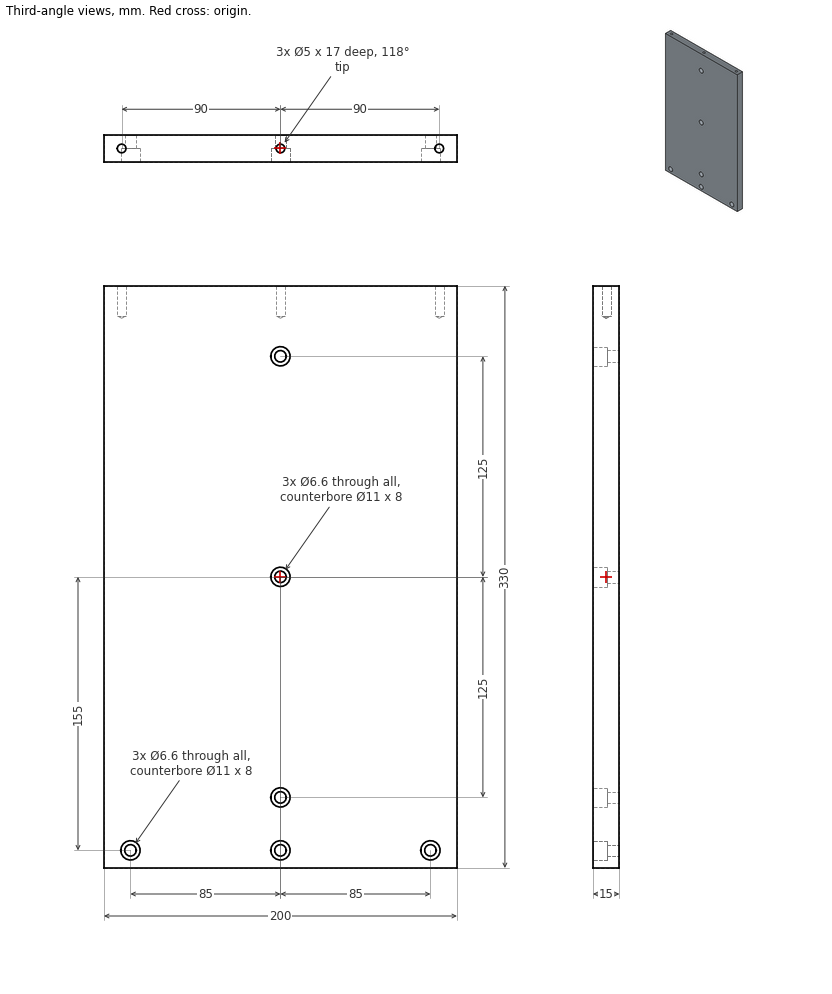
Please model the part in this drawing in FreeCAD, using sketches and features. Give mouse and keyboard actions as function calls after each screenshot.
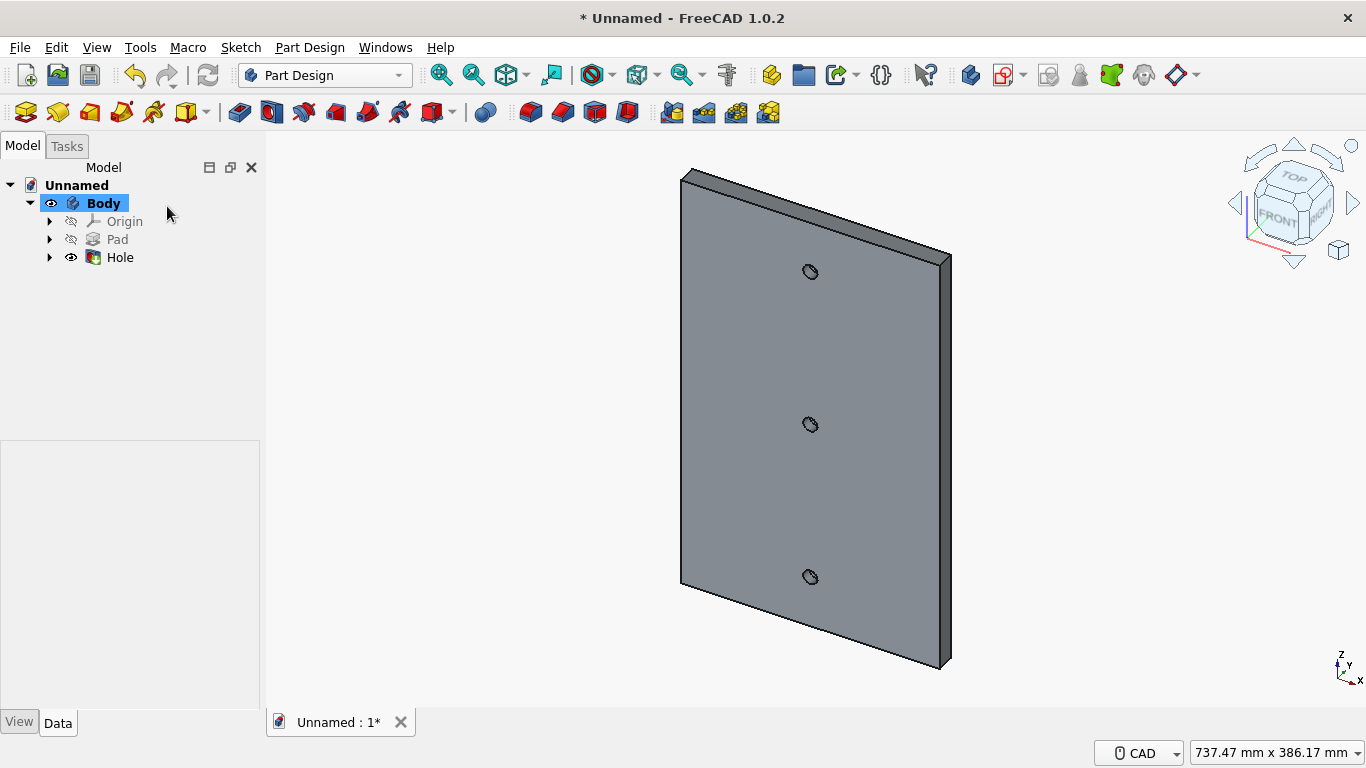
click(847, 493)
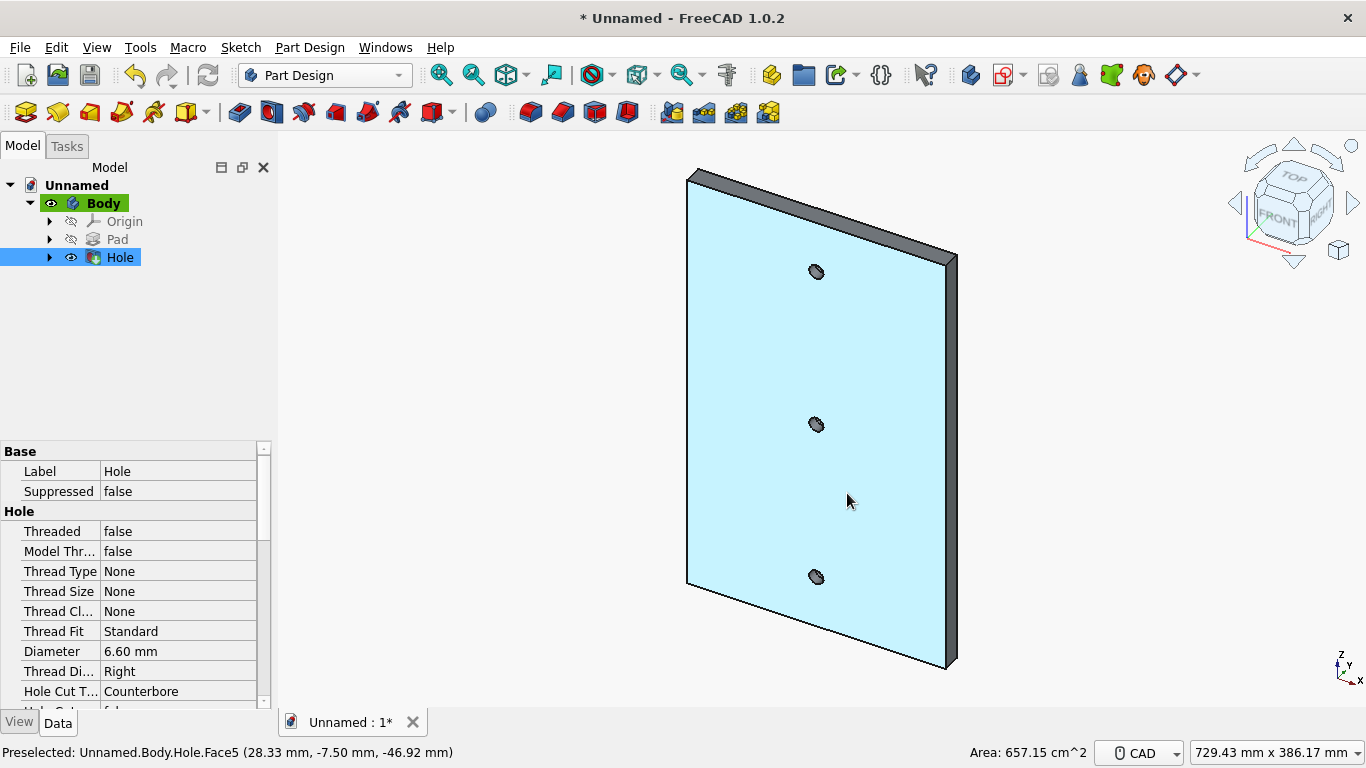
click(1004, 76)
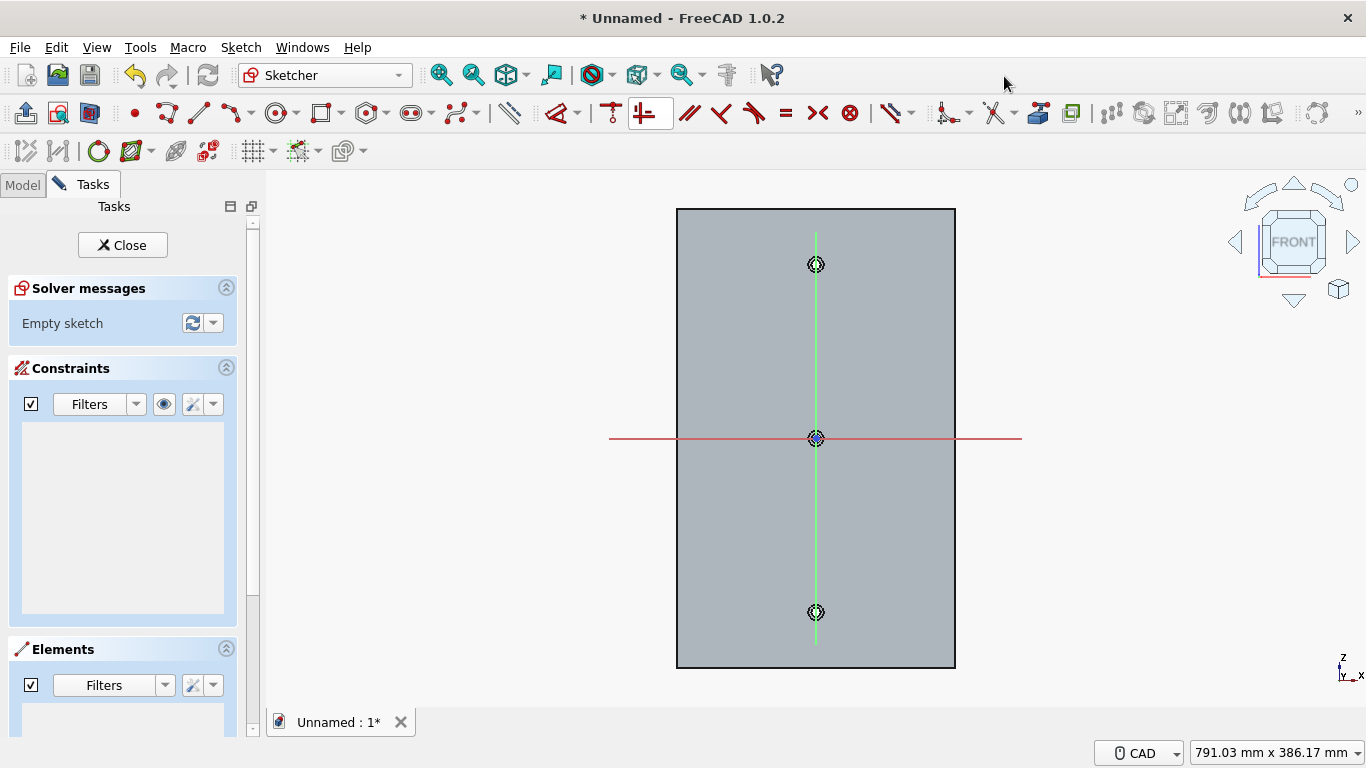
scroll(955, 679, up, 2)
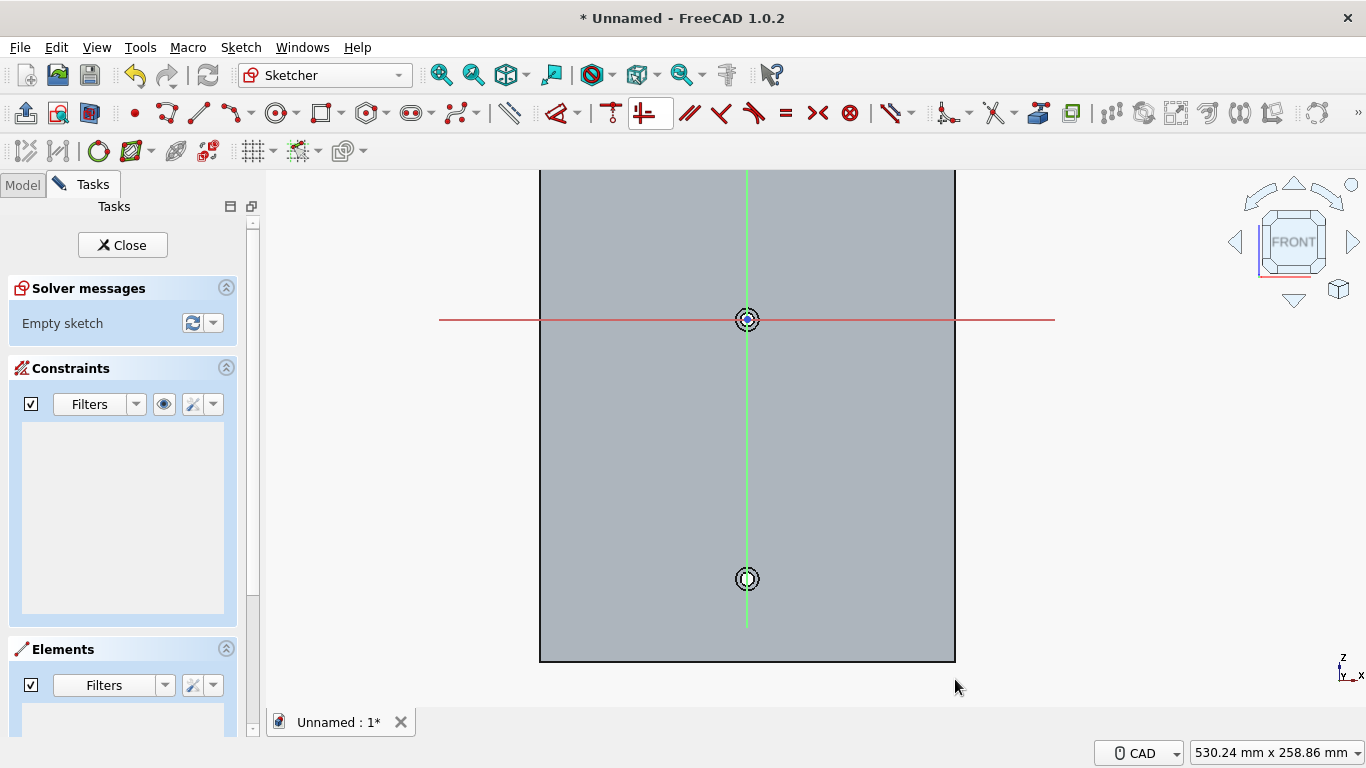
key(g)
key(c)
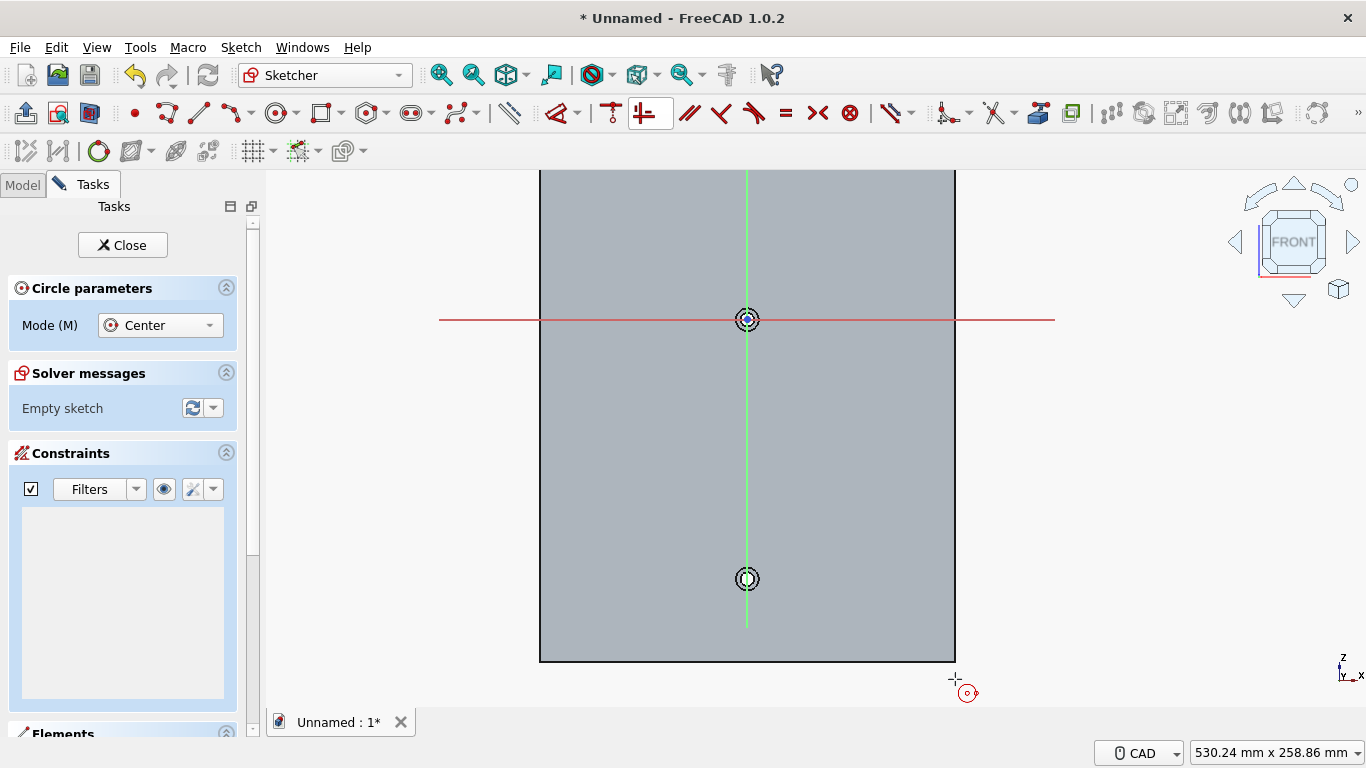
scroll(571, 641, up, 6)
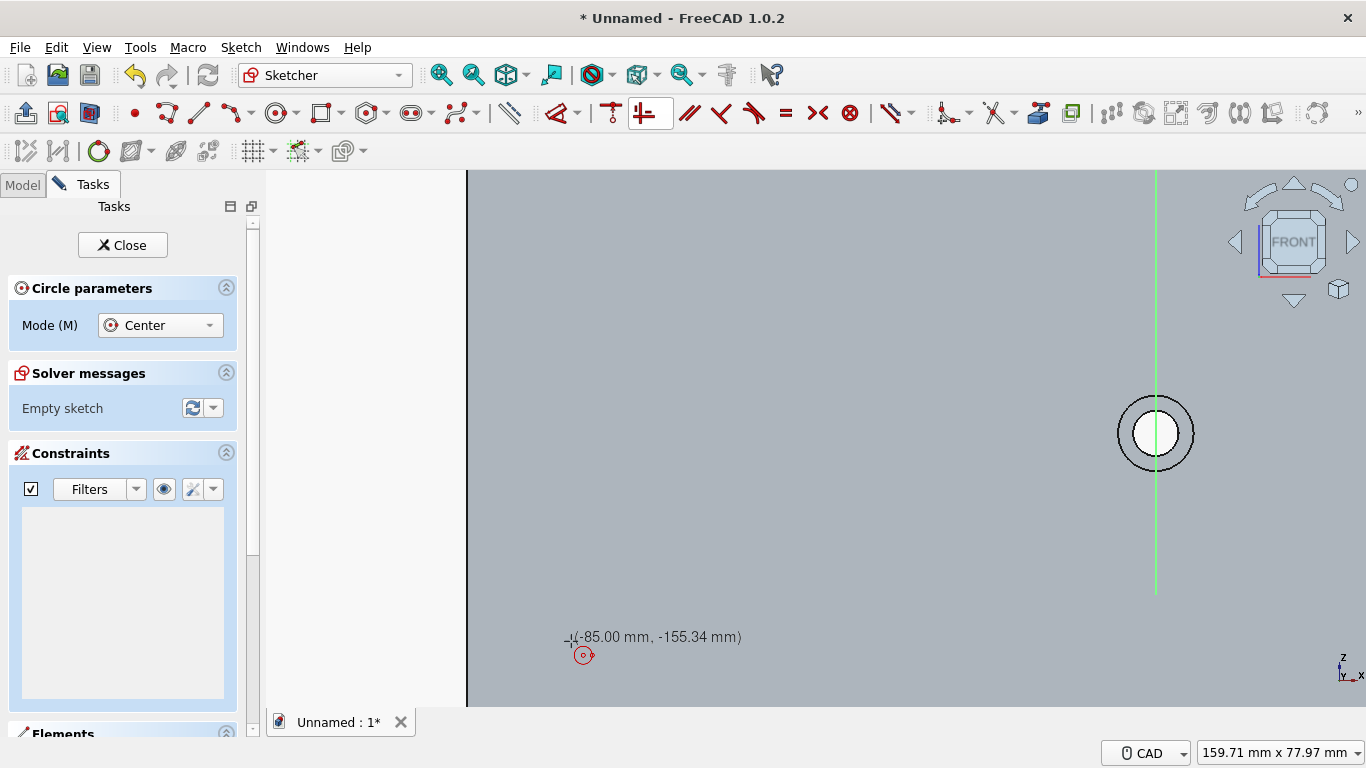
click(570, 640)
click(586, 624)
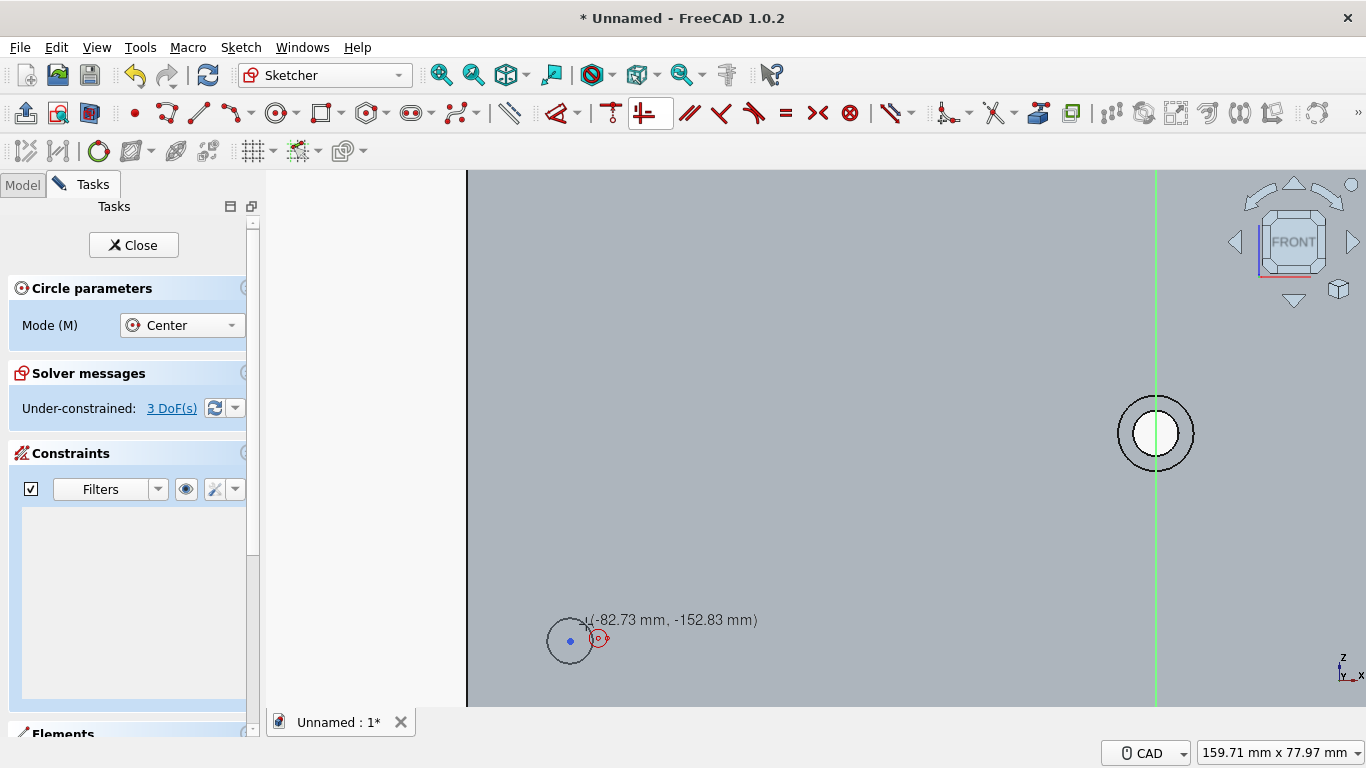
click(1156, 640)
click(1172, 624)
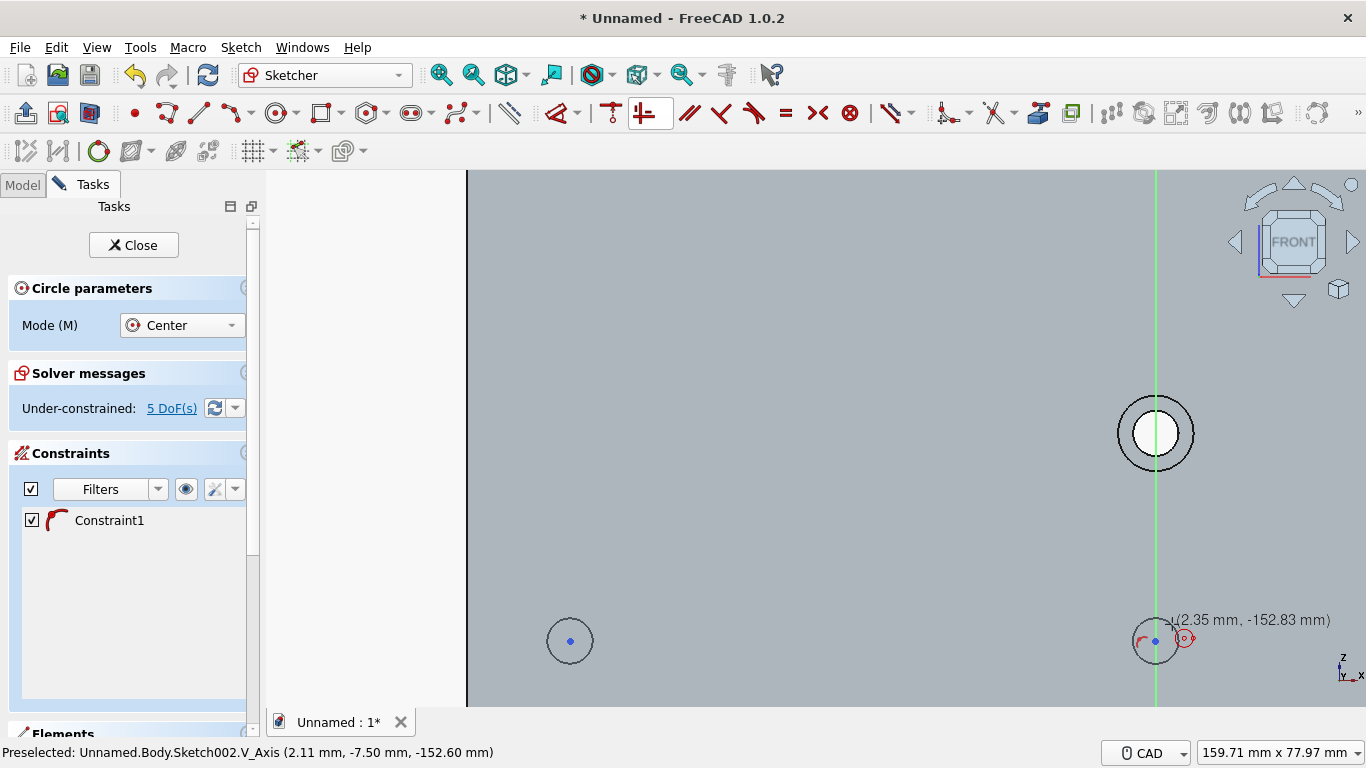
scroll(572, 577, down, 6)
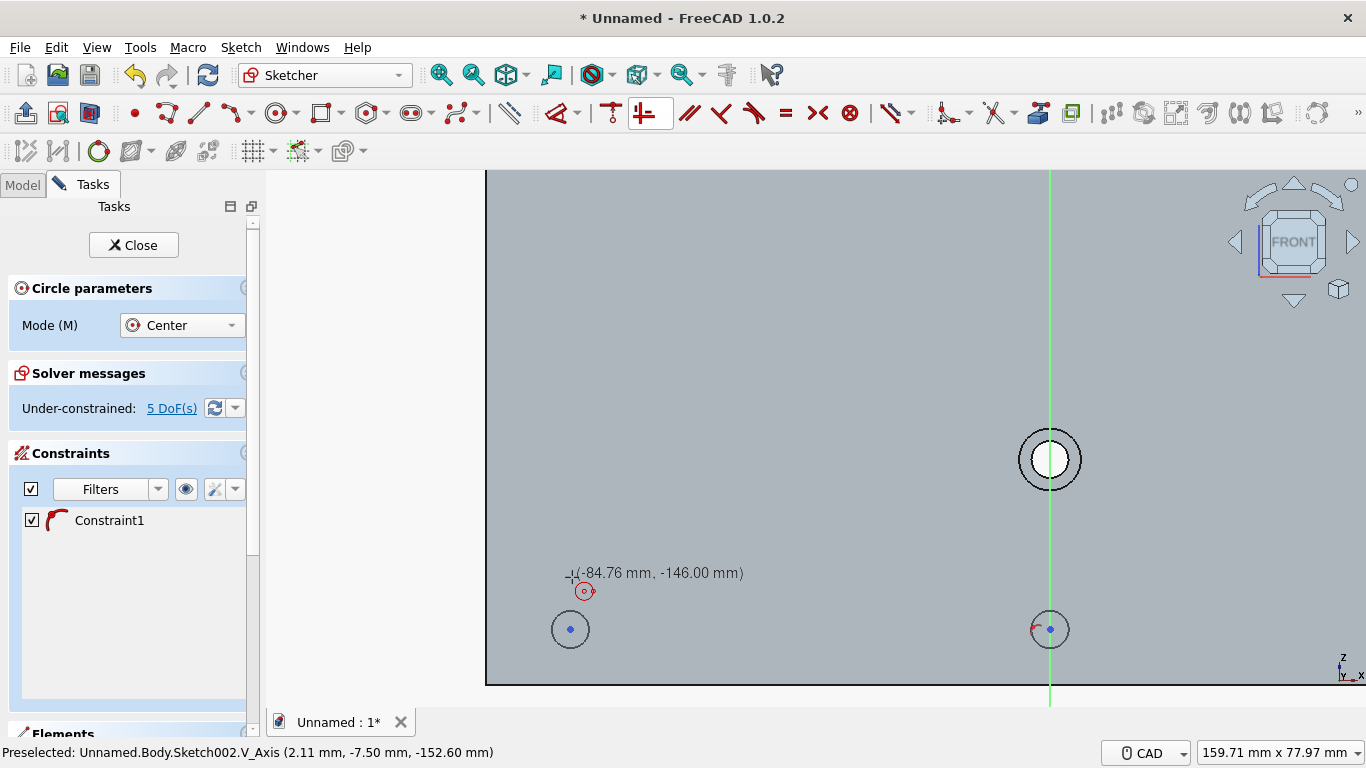
scroll(924, 596, up, 6)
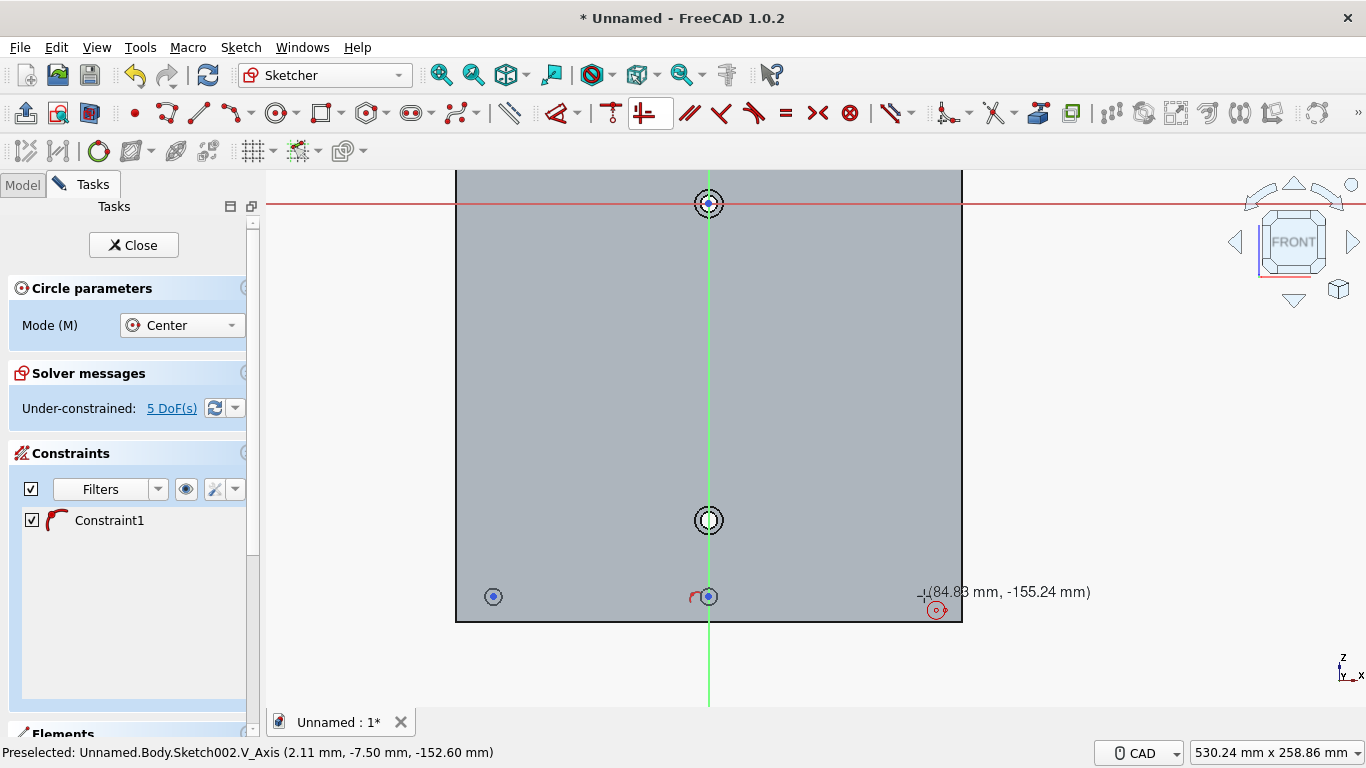
click(924, 596)
click(940, 580)
key(Escape)